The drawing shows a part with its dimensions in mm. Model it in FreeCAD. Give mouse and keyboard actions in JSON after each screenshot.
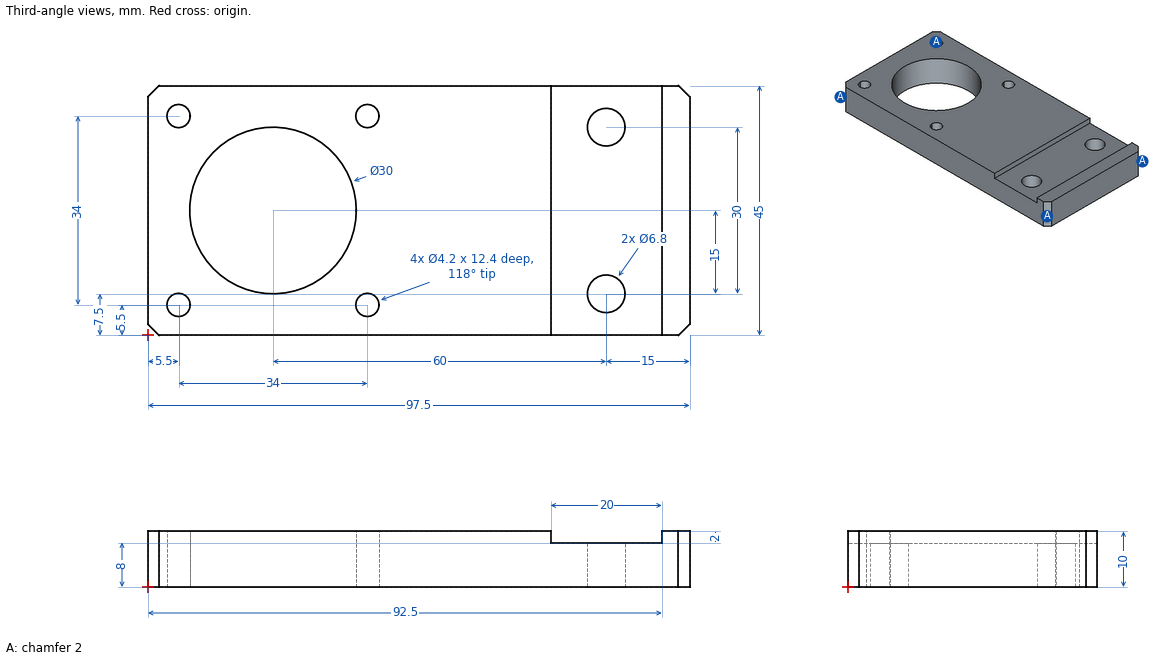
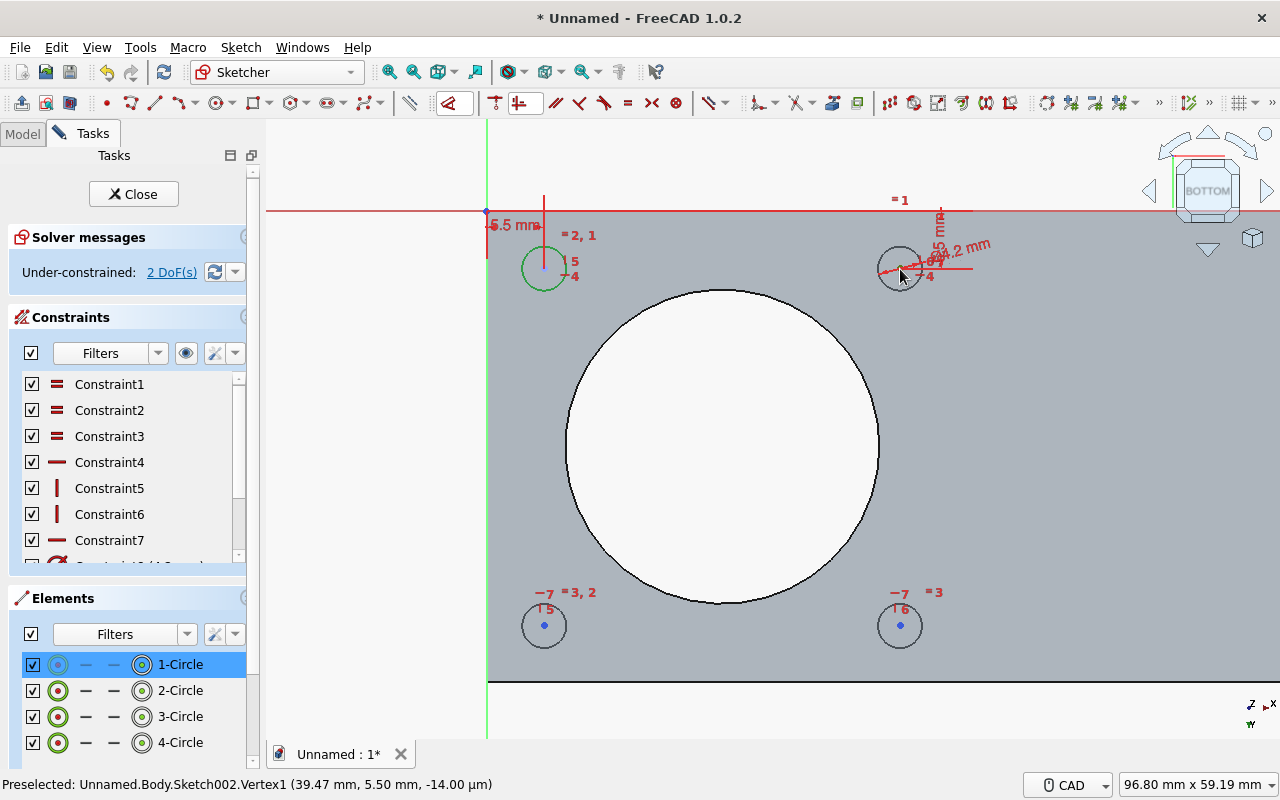
{"action": "left_click", "coordinate": [544, 269]}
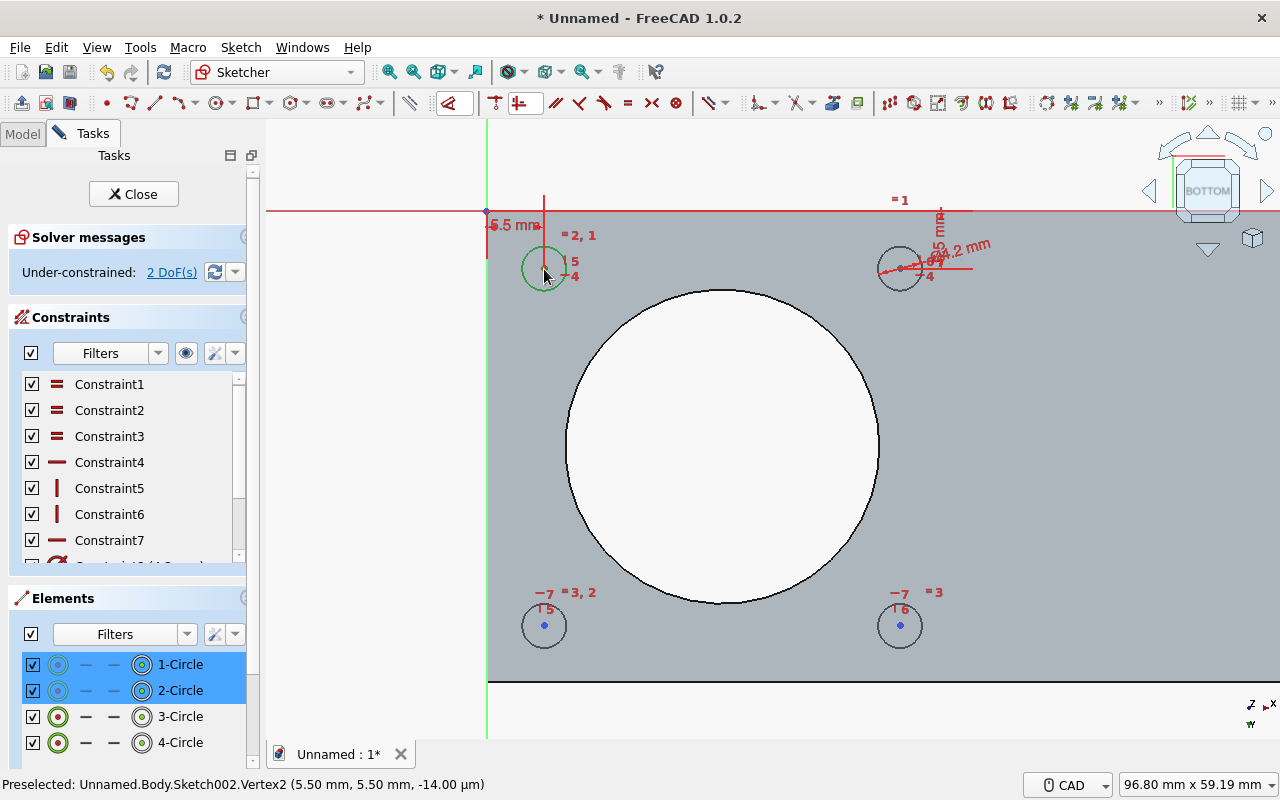
{"action": "key", "text": "l"}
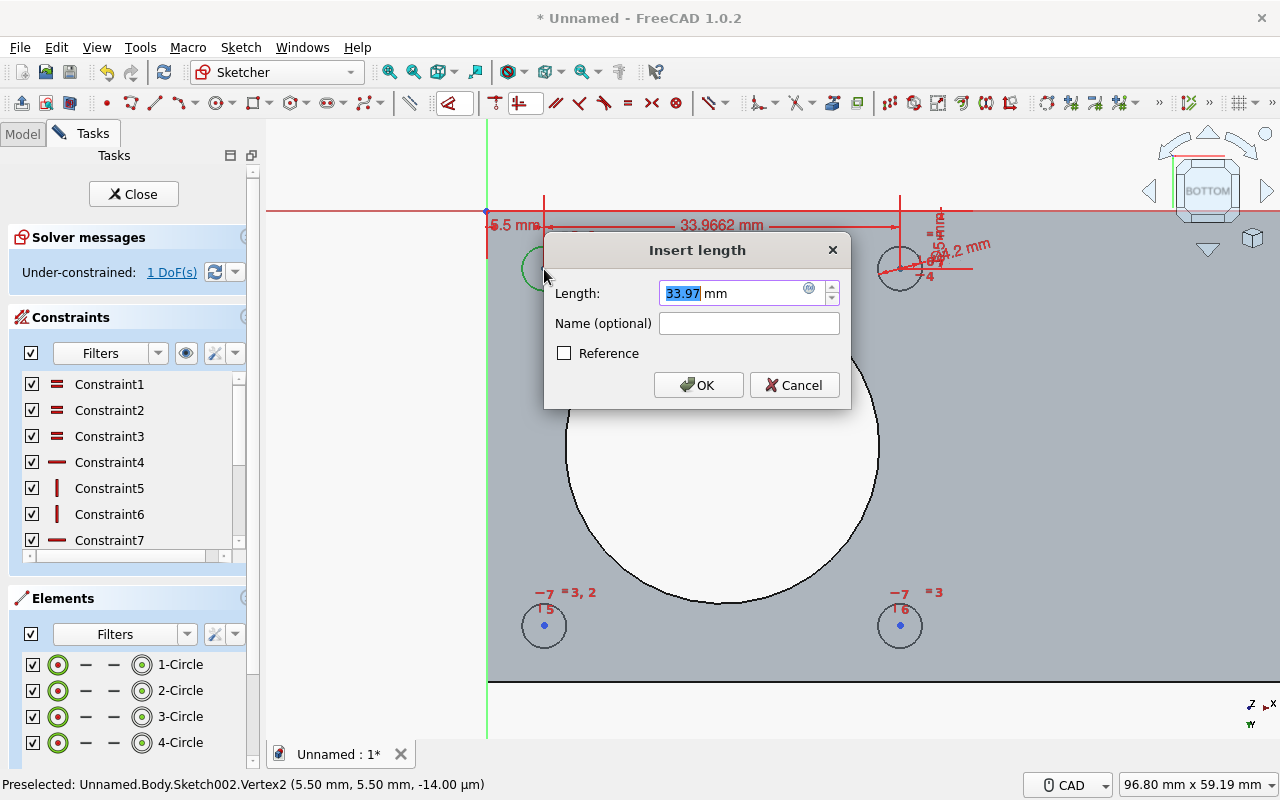
{"action": "type", "text": "34"}
{"action": "key", "text": "Return"}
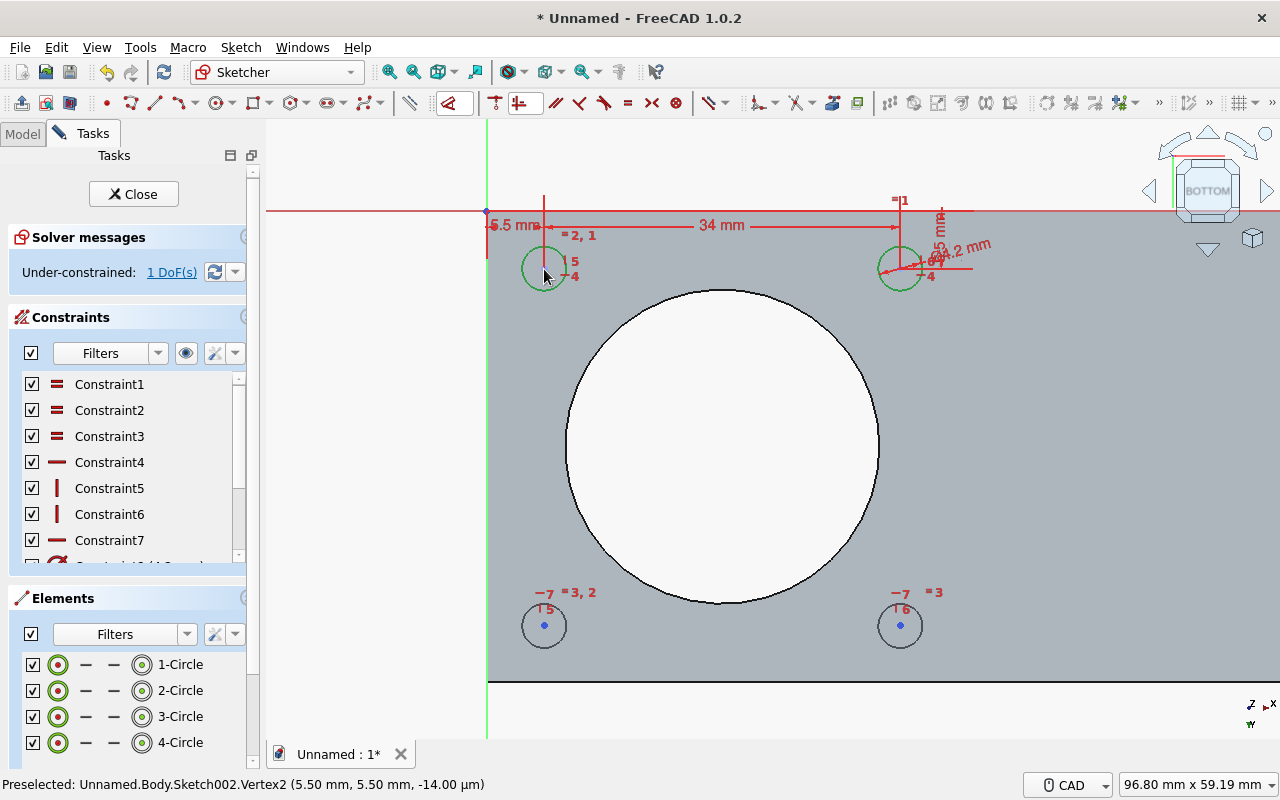
{"action": "left_click", "coordinate": [544, 269]}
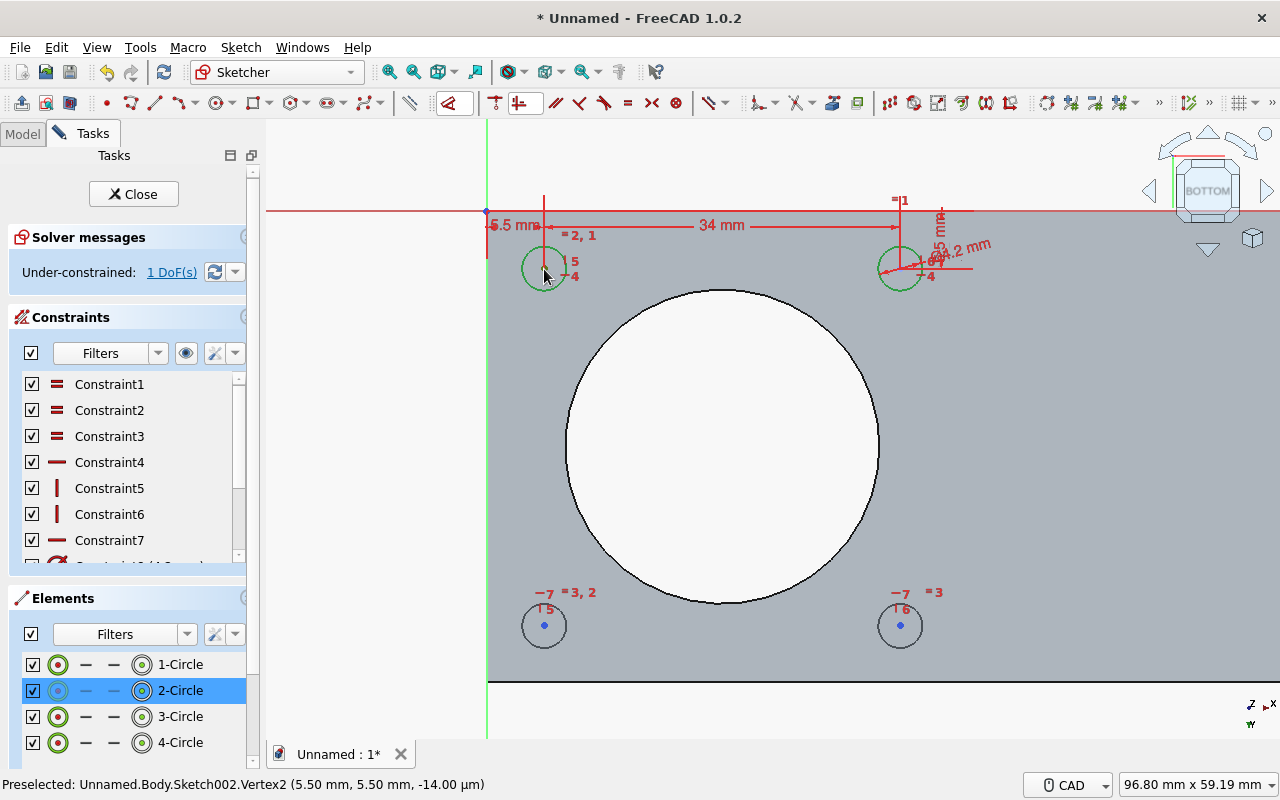
{"action": "left_click", "coordinate": [544, 626]}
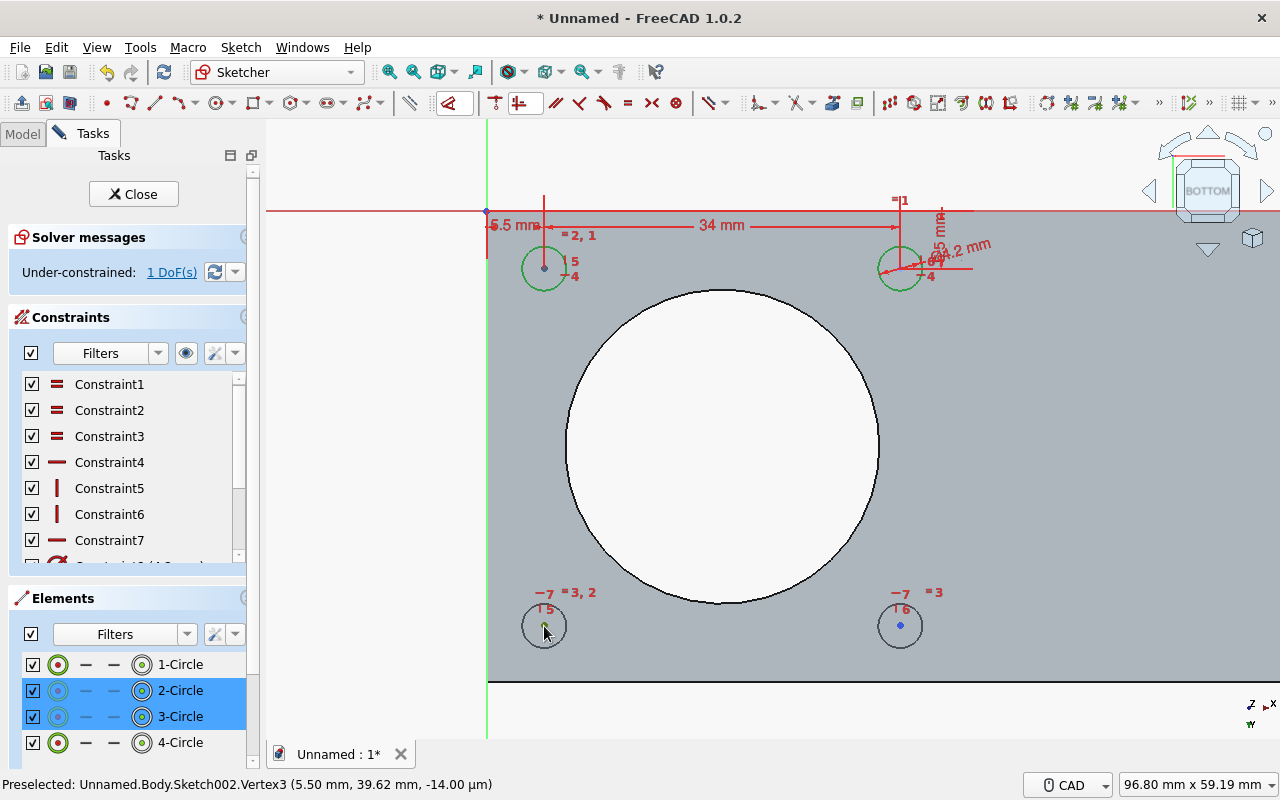
{"action": "key", "text": "i"}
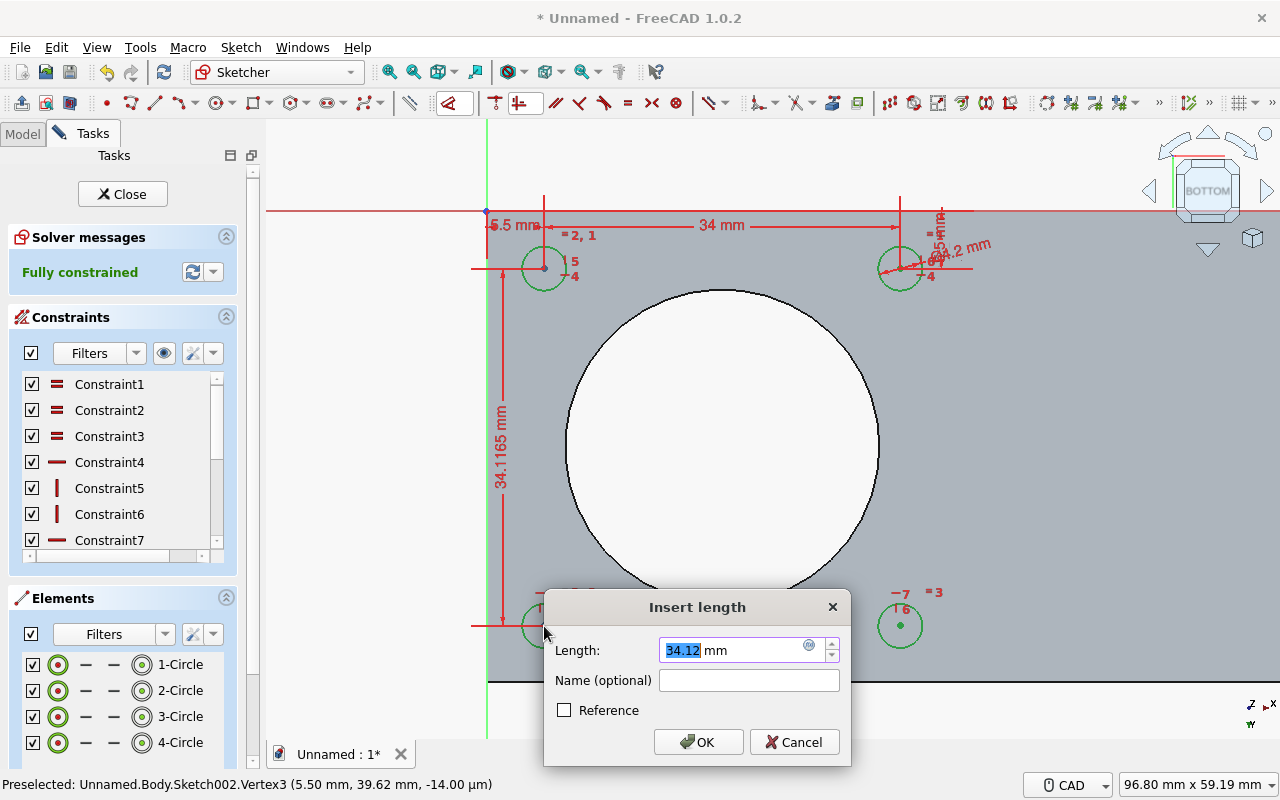
{"action": "type", "text": "34"}
{"action": "key", "text": "Return"}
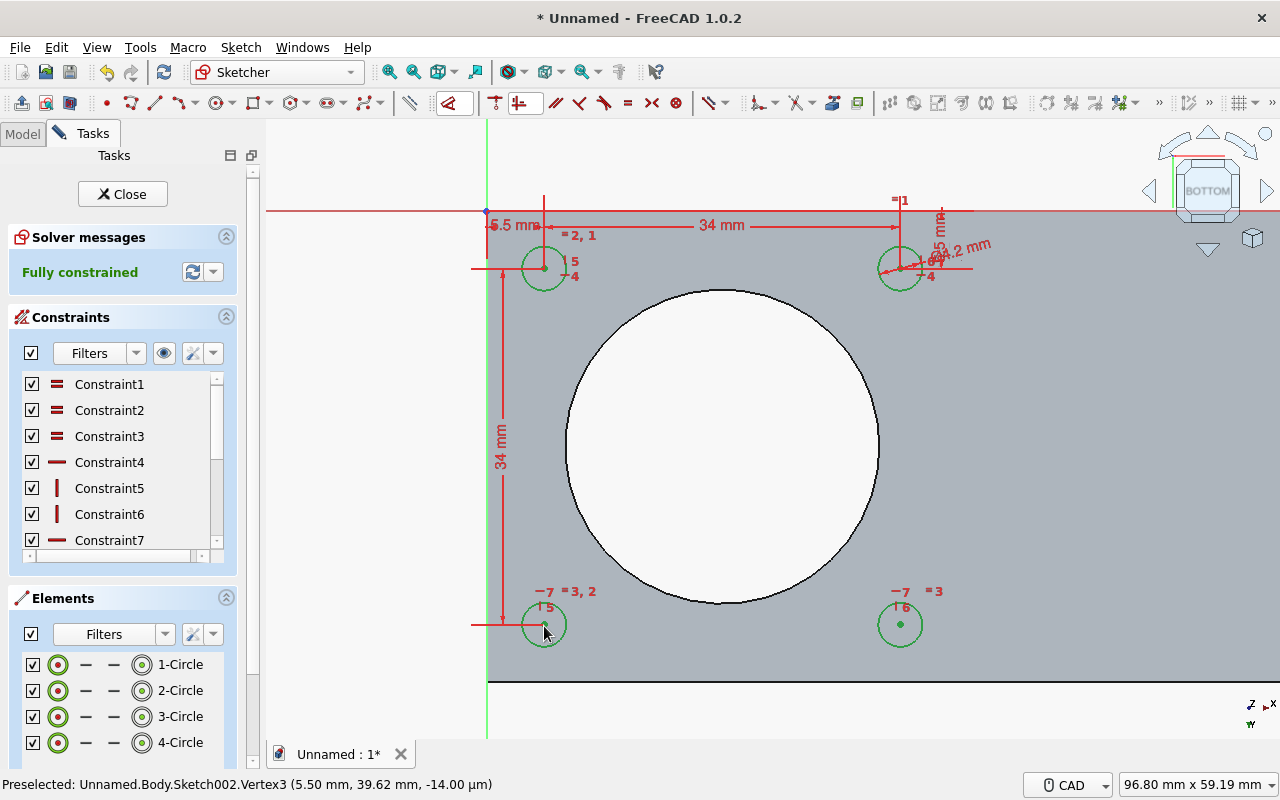
{"action": "left_click", "coordinate": [123, 194]}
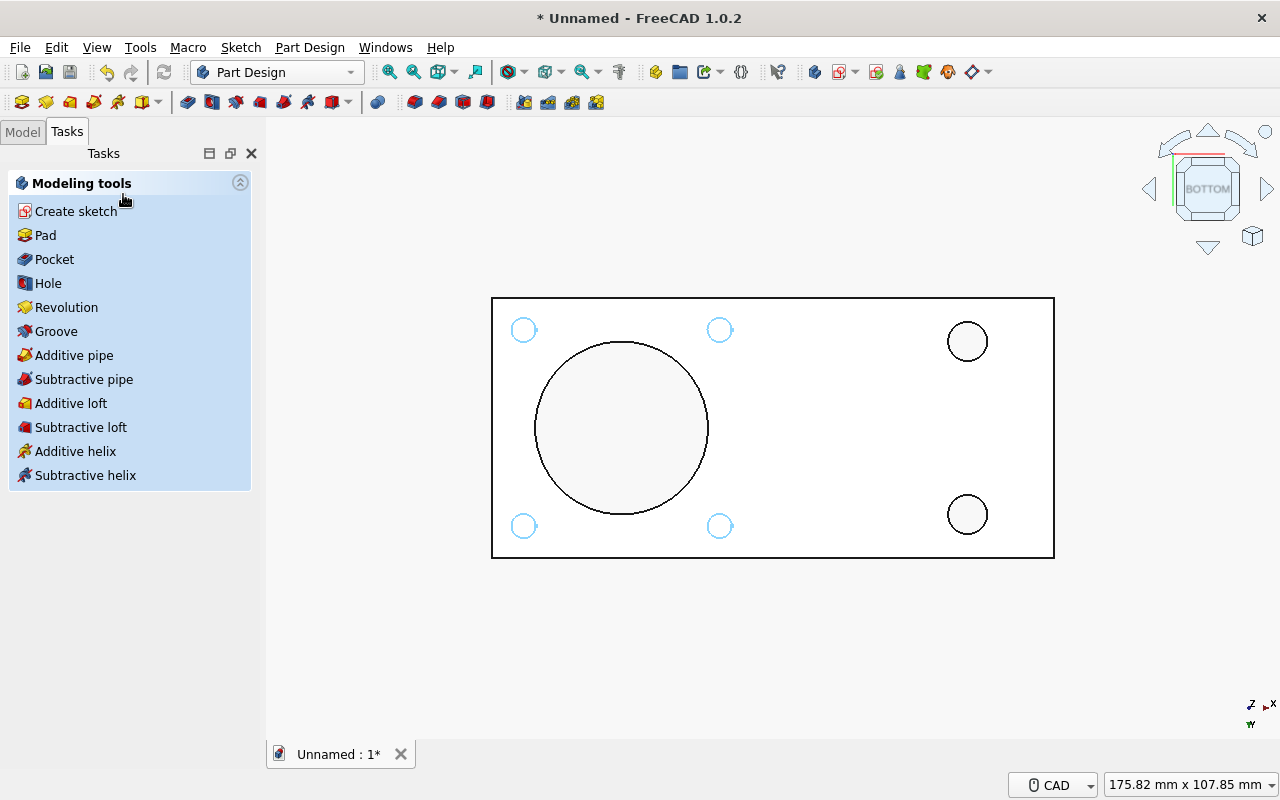
{"action": "left_click", "coordinate": [212, 102]}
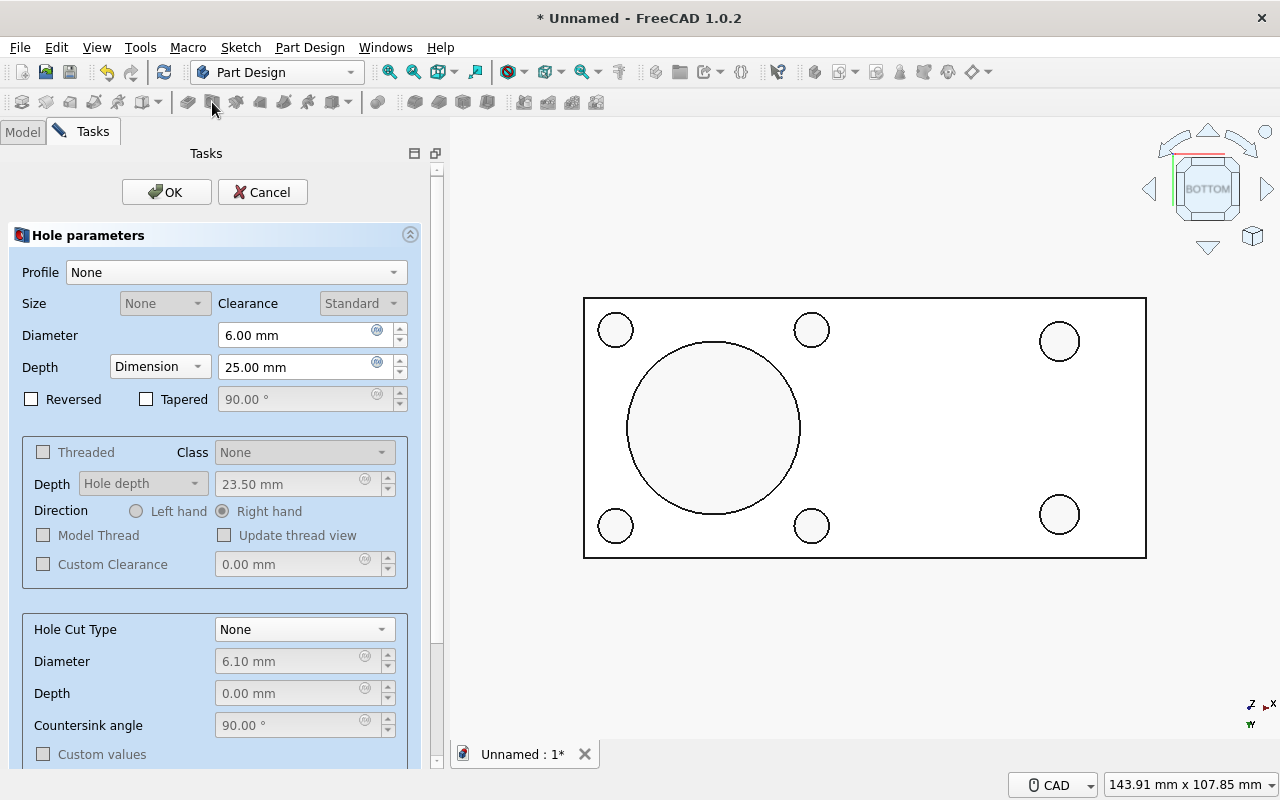
{"action": "triple_click", "coordinate": [305, 335]}